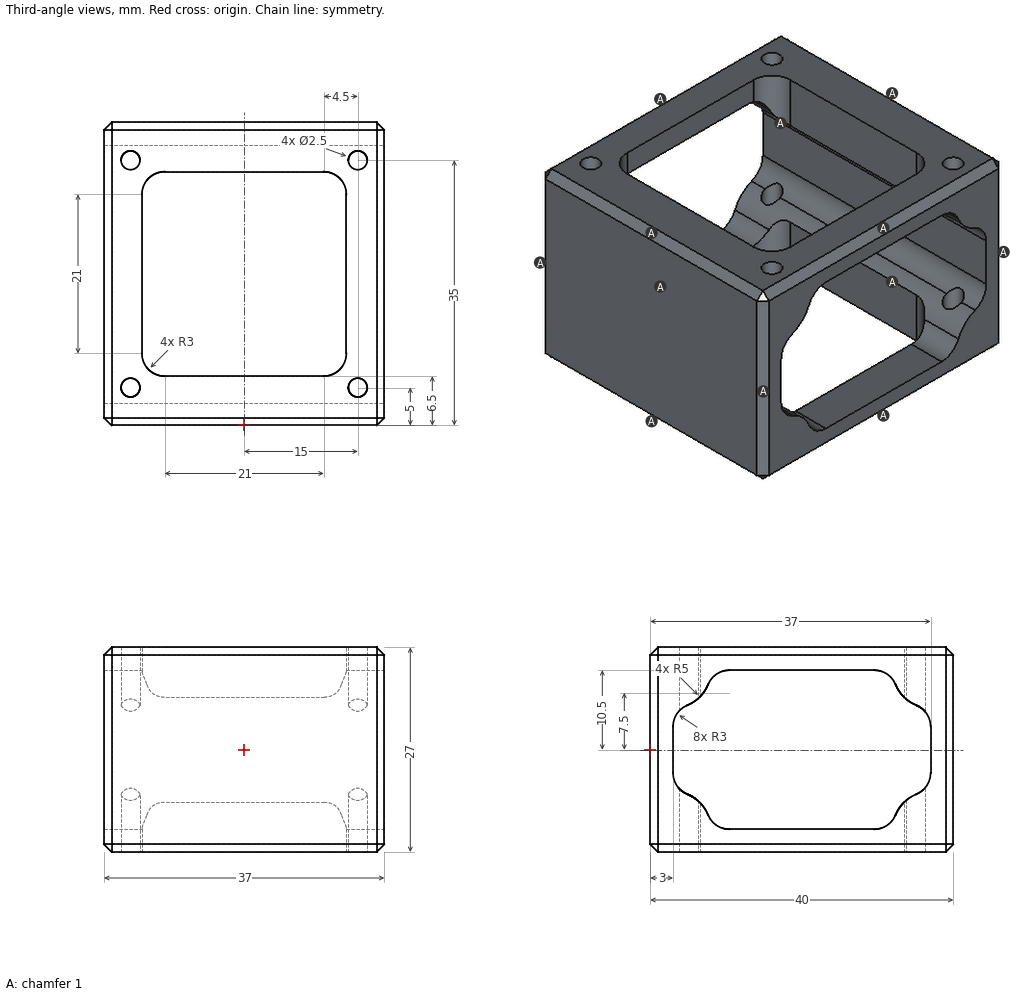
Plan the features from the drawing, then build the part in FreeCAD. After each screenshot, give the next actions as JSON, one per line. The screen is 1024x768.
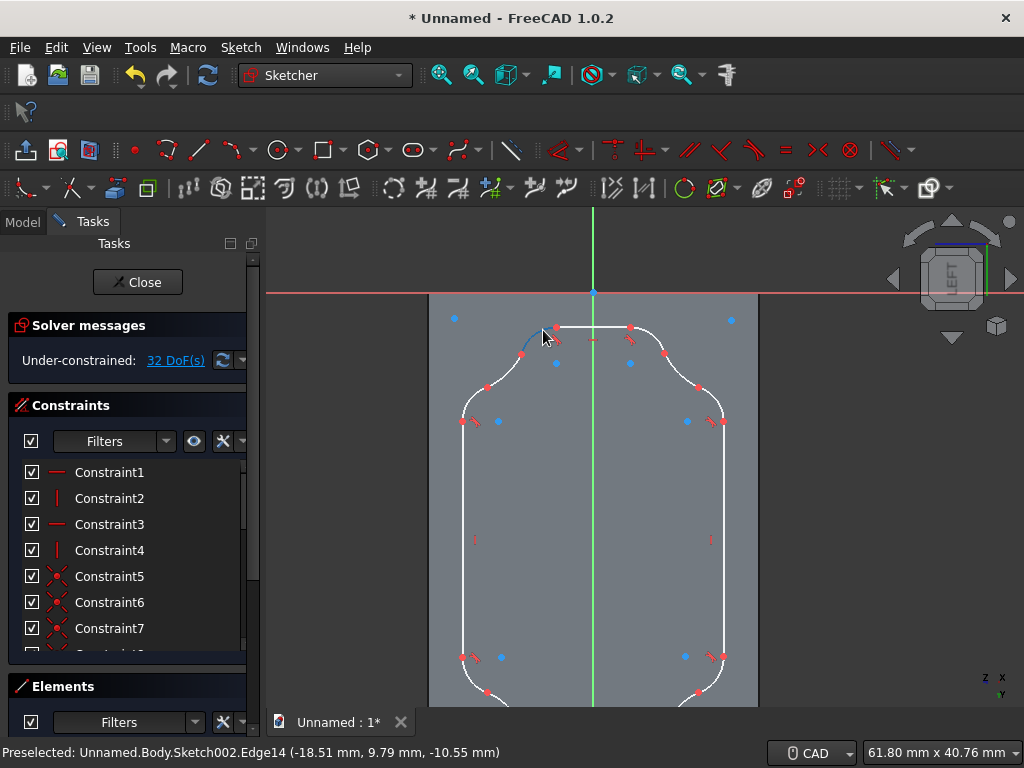
{"action": "left_click", "coordinate": [542, 330]}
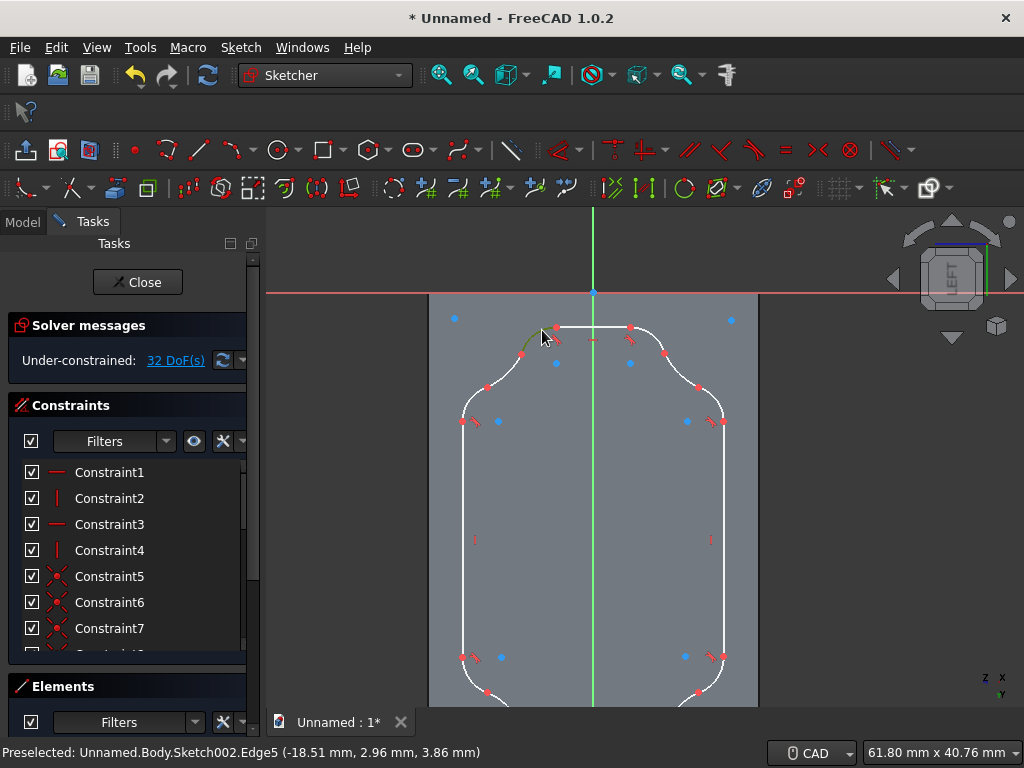
{"action": "left_click", "coordinate": [500, 380]}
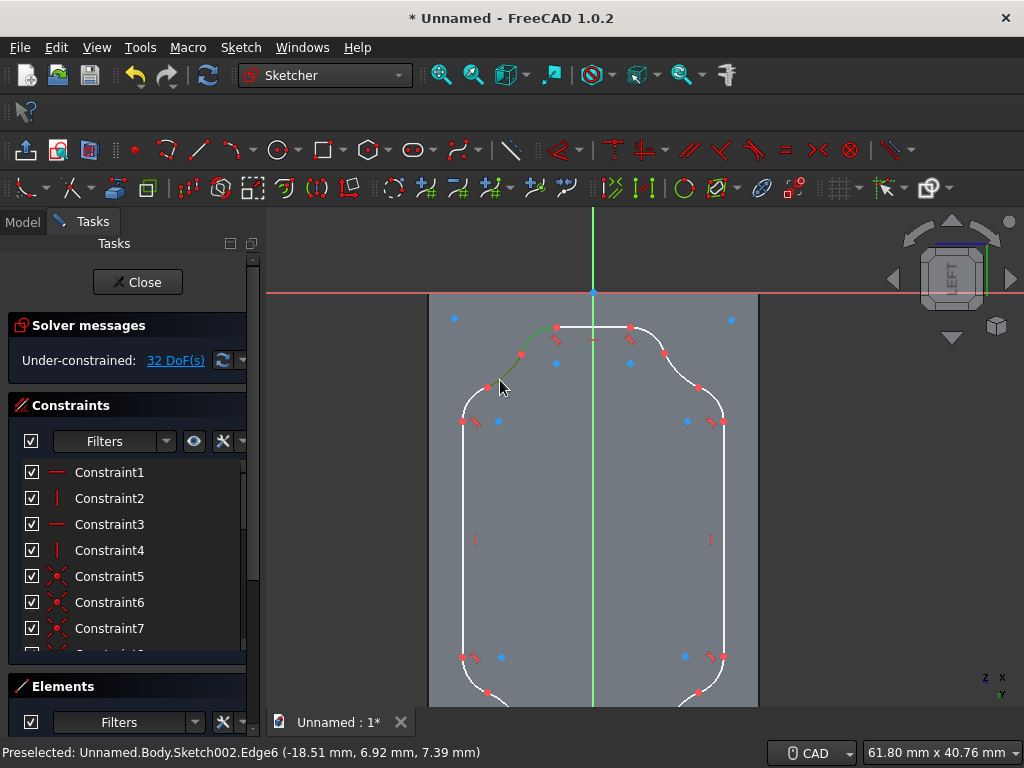
{"action": "left_click", "coordinate": [754, 150]}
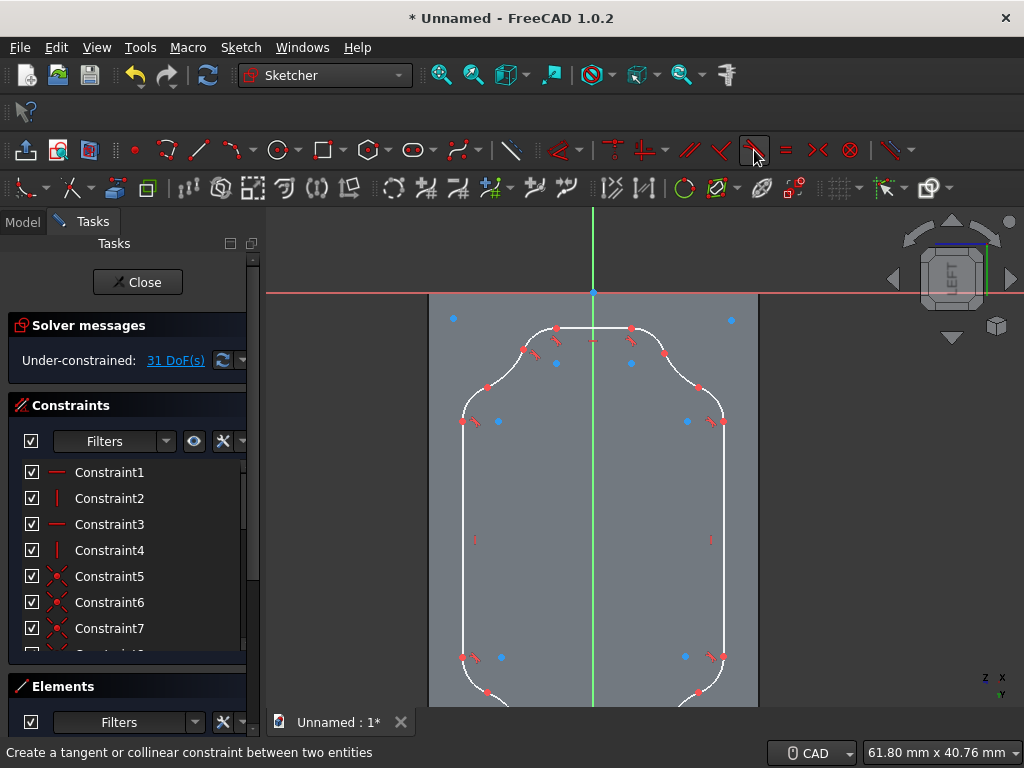
{"action": "left_click", "coordinate": [501, 379]}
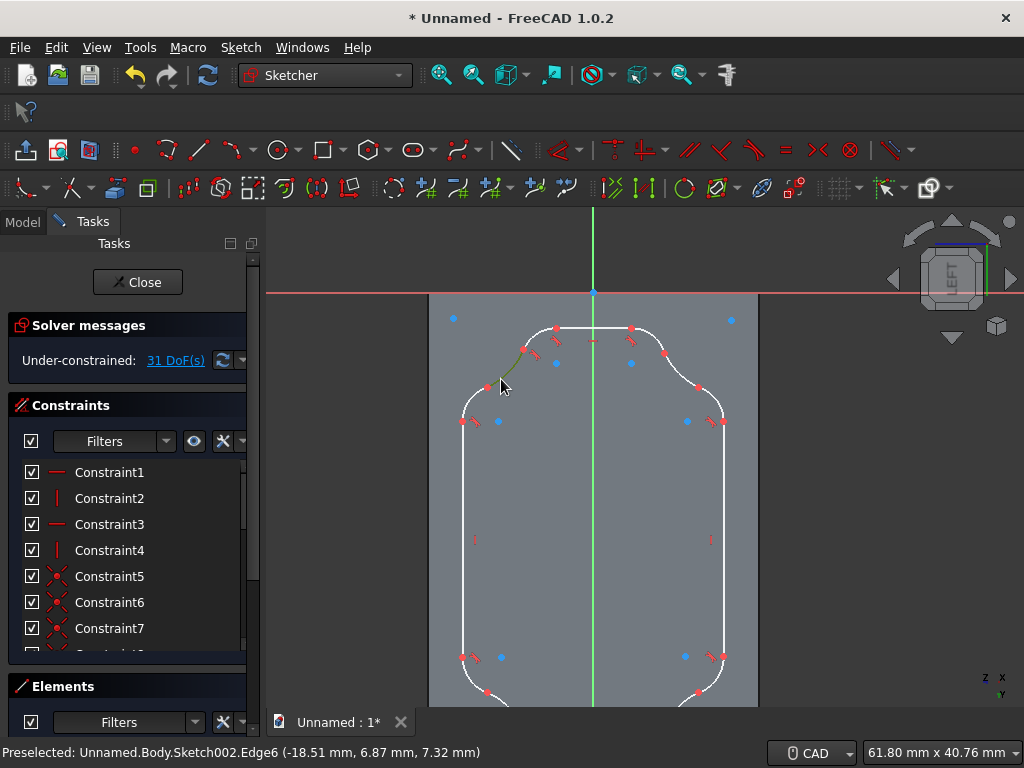
{"action": "left_click", "coordinate": [475, 394]}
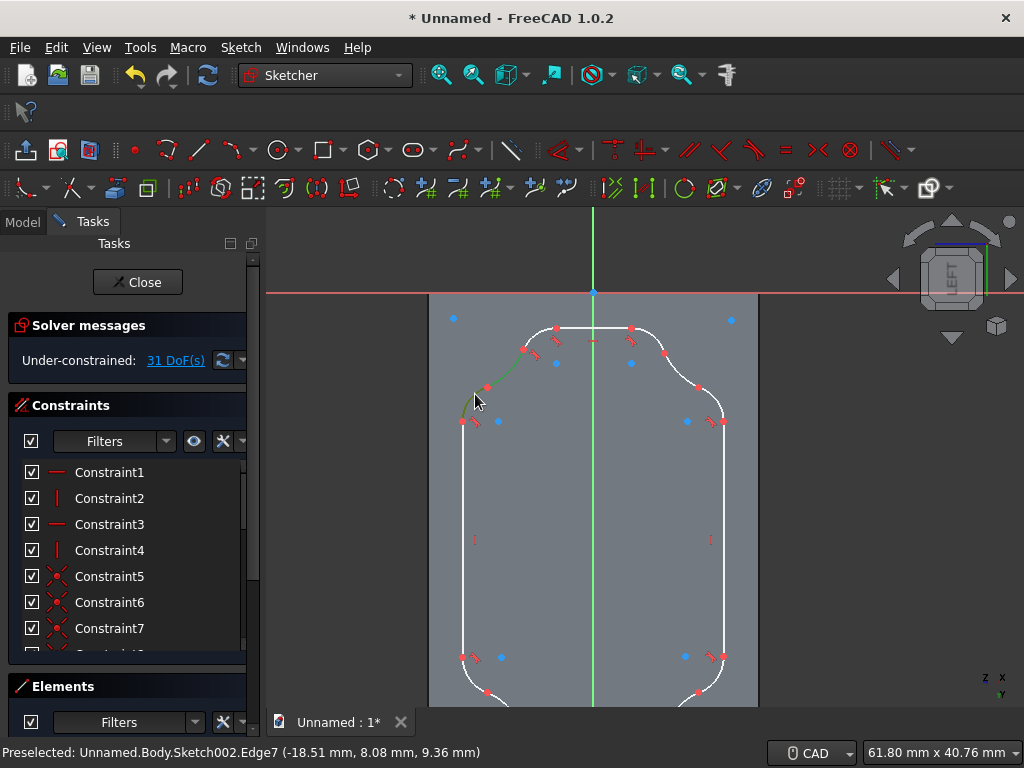
{"action": "key", "text": "t"}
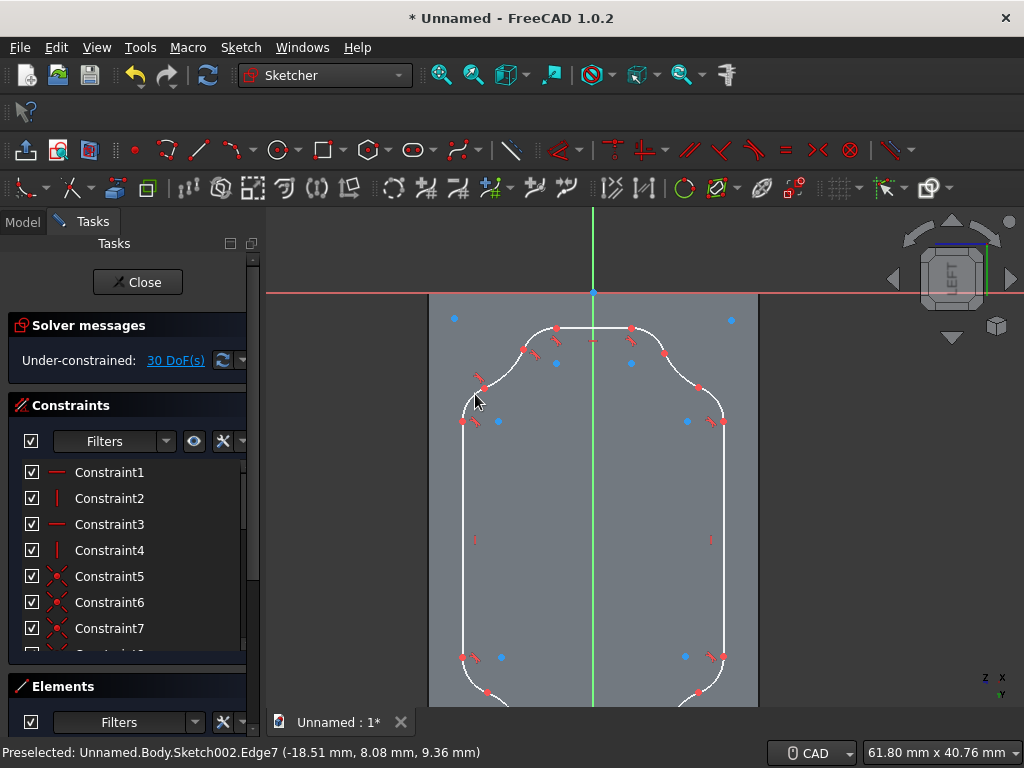
{"action": "left_click", "coordinate": [465, 671]}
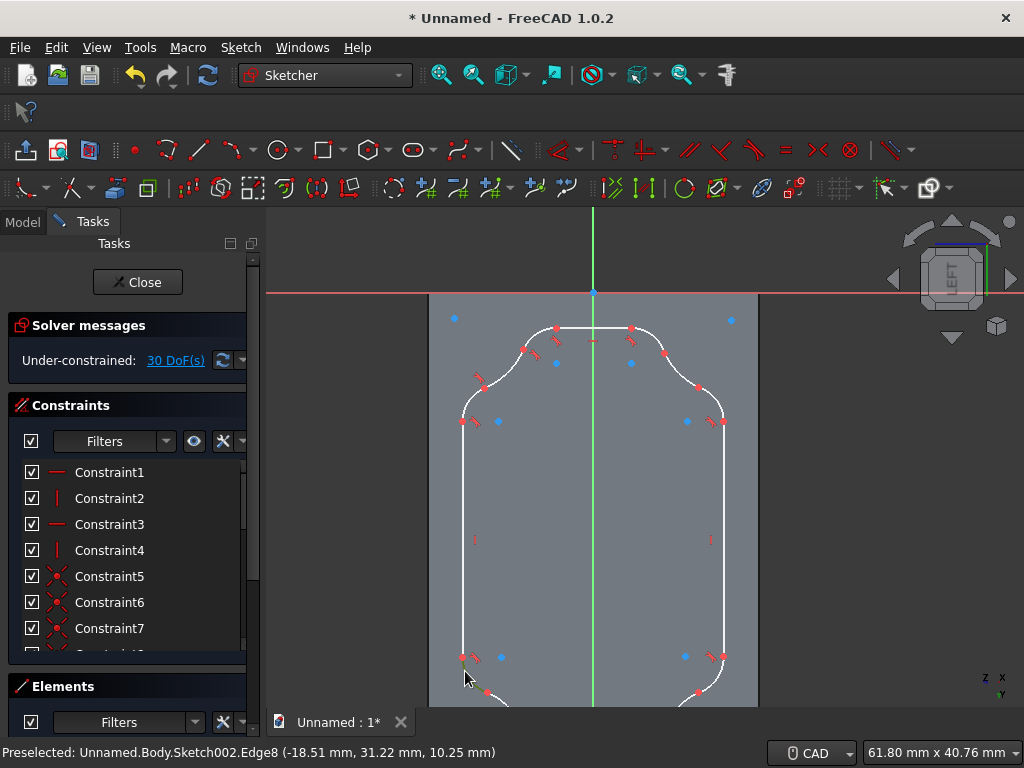
{"action": "scroll", "coordinate": [543, 330], "scroll_direction": "down", "scroll_amount": 2}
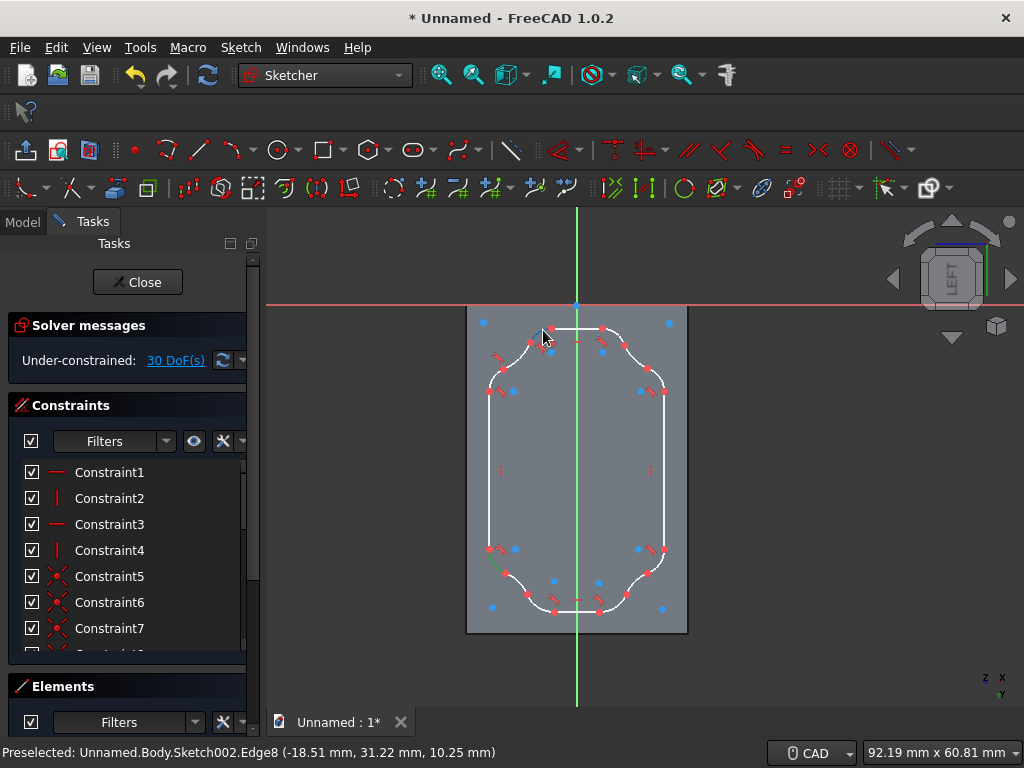
{"action": "scroll", "coordinate": [523, 586], "scroll_direction": "up", "scroll_amount": 2}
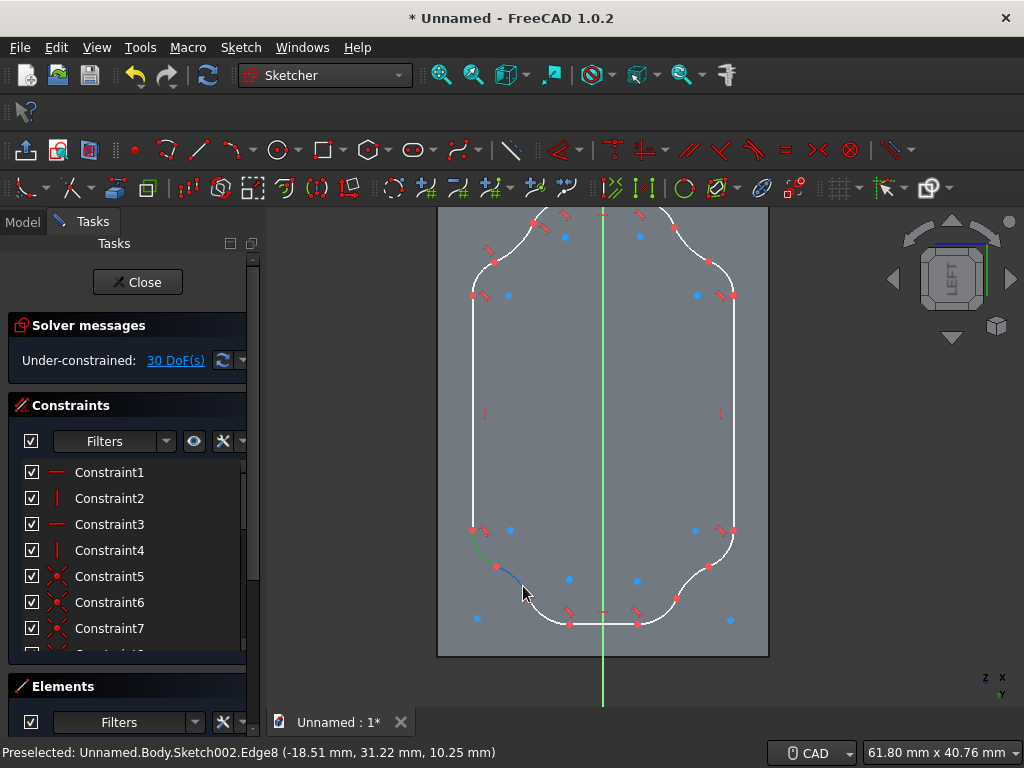
{"action": "left_click", "coordinate": [522, 586]}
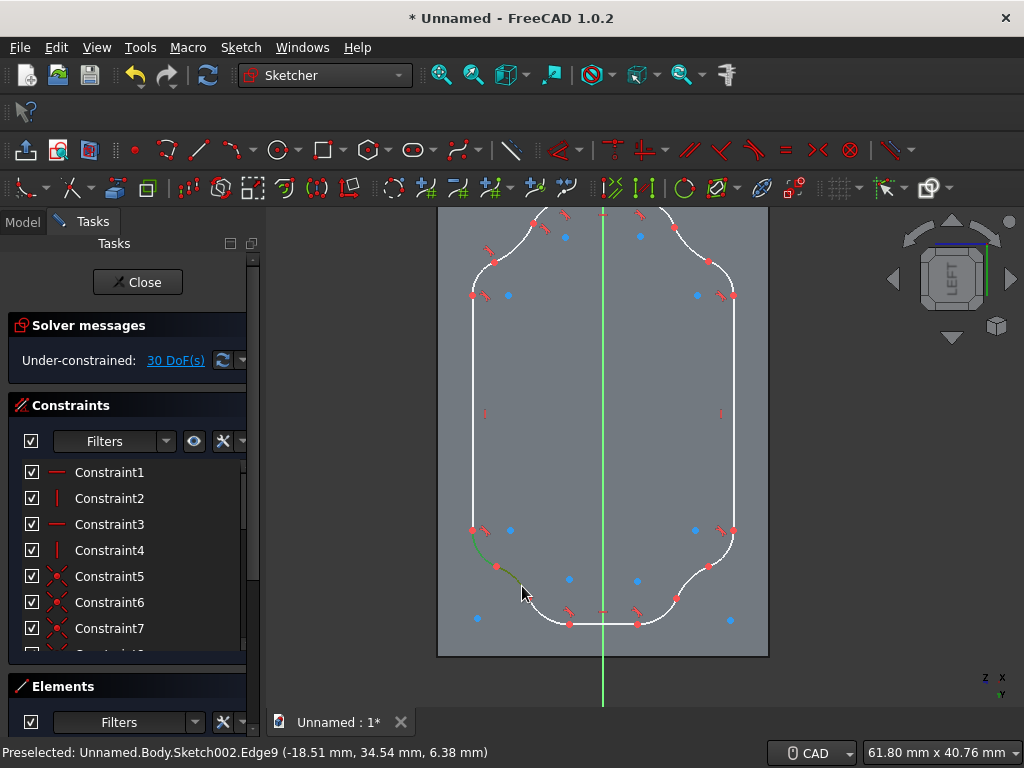
{"action": "left_click", "coordinate": [754, 150]}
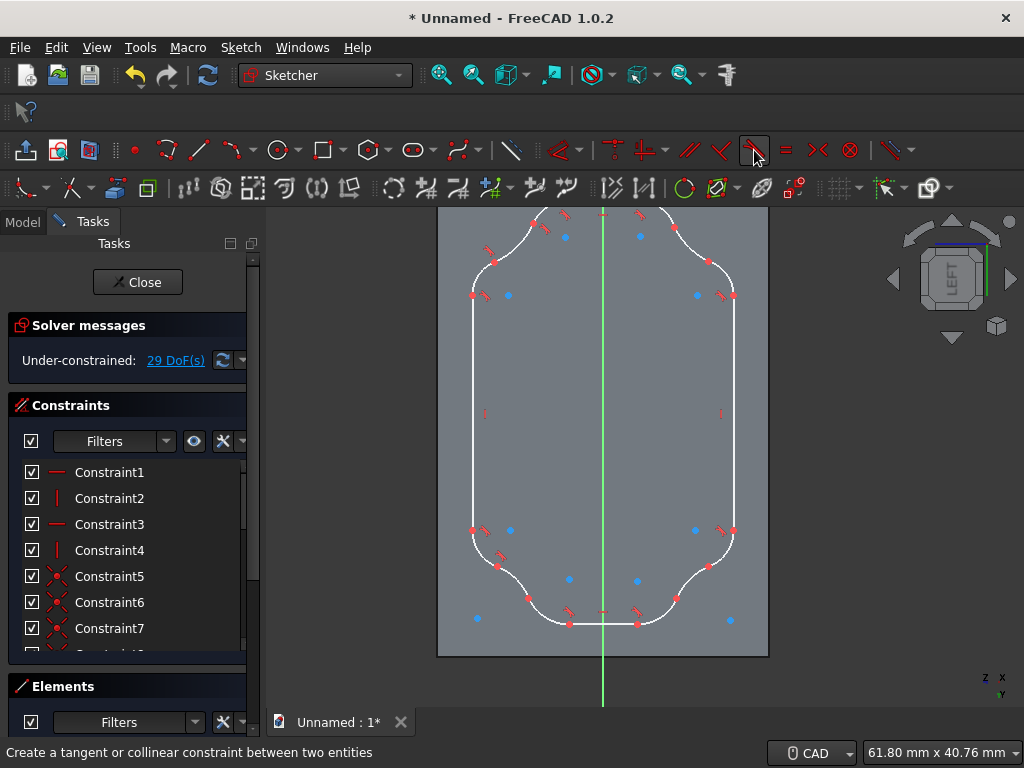
{"action": "left_click", "coordinate": [522, 586]}